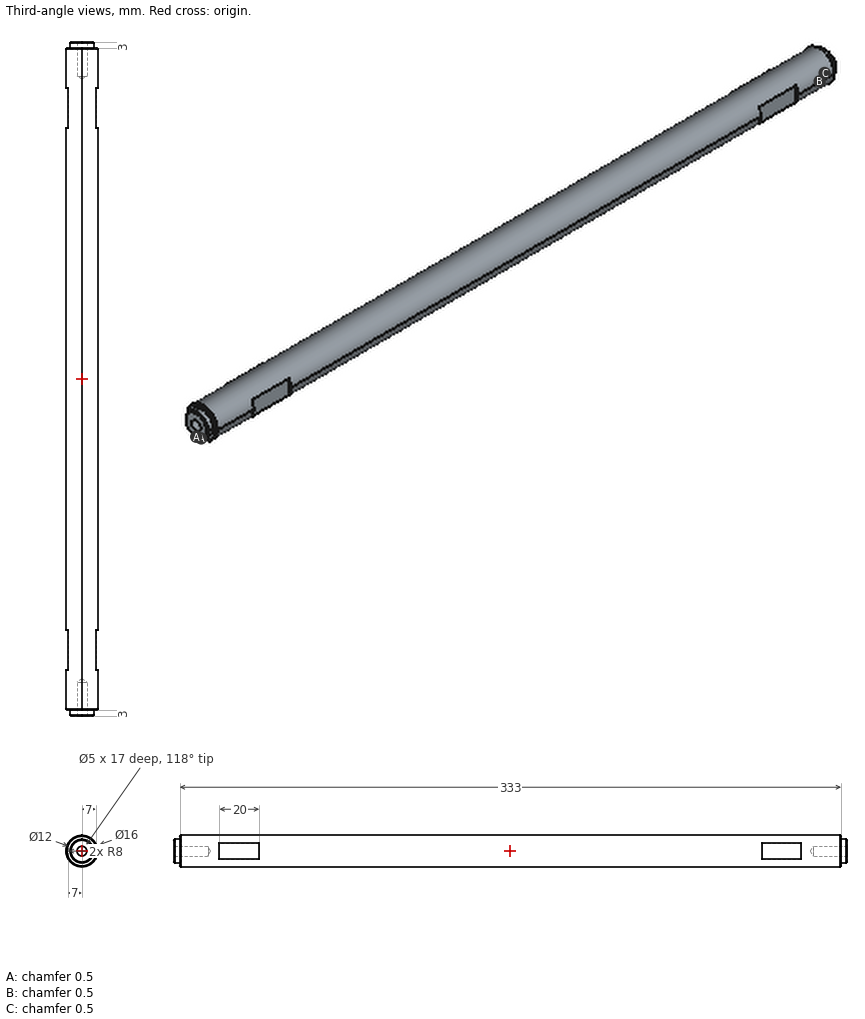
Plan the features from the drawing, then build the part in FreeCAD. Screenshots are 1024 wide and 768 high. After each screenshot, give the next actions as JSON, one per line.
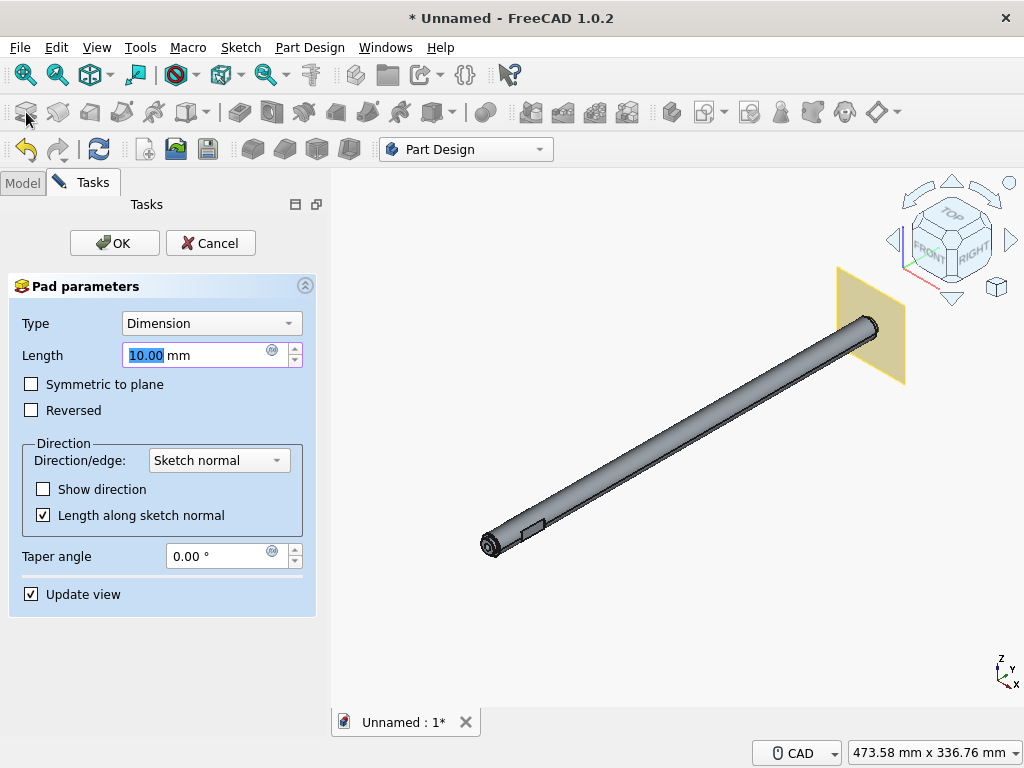
{"action": "type", "text": "3"}
{"action": "key", "text": "Tab"}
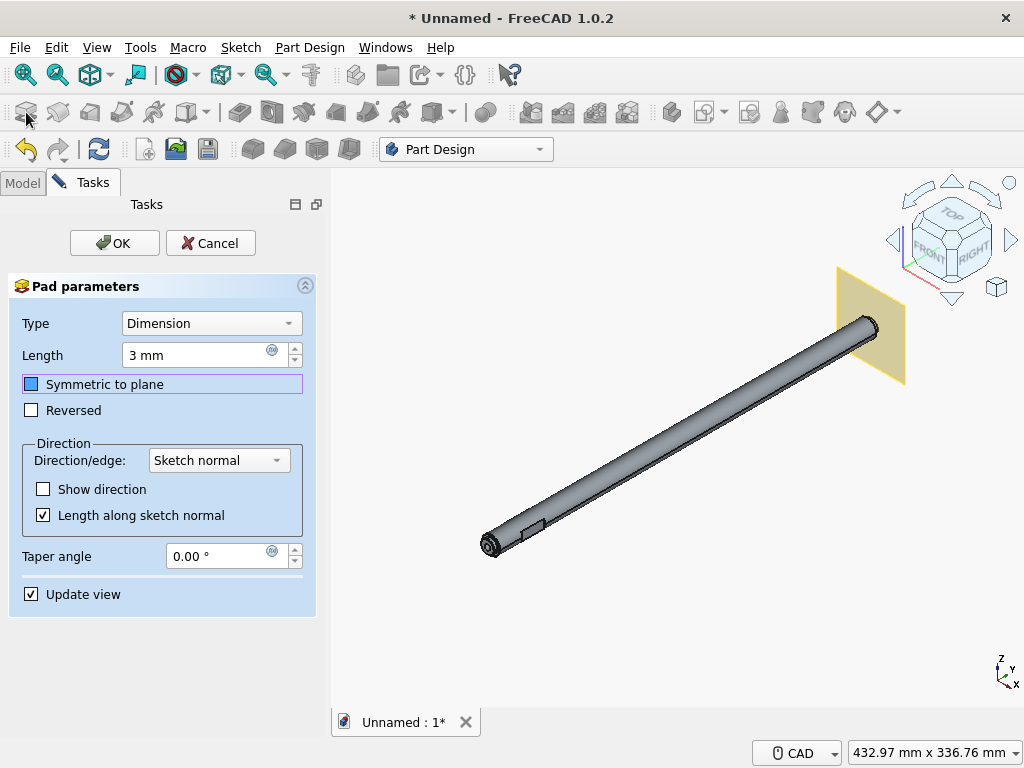
{"action": "left_click", "coordinate": [115, 243]}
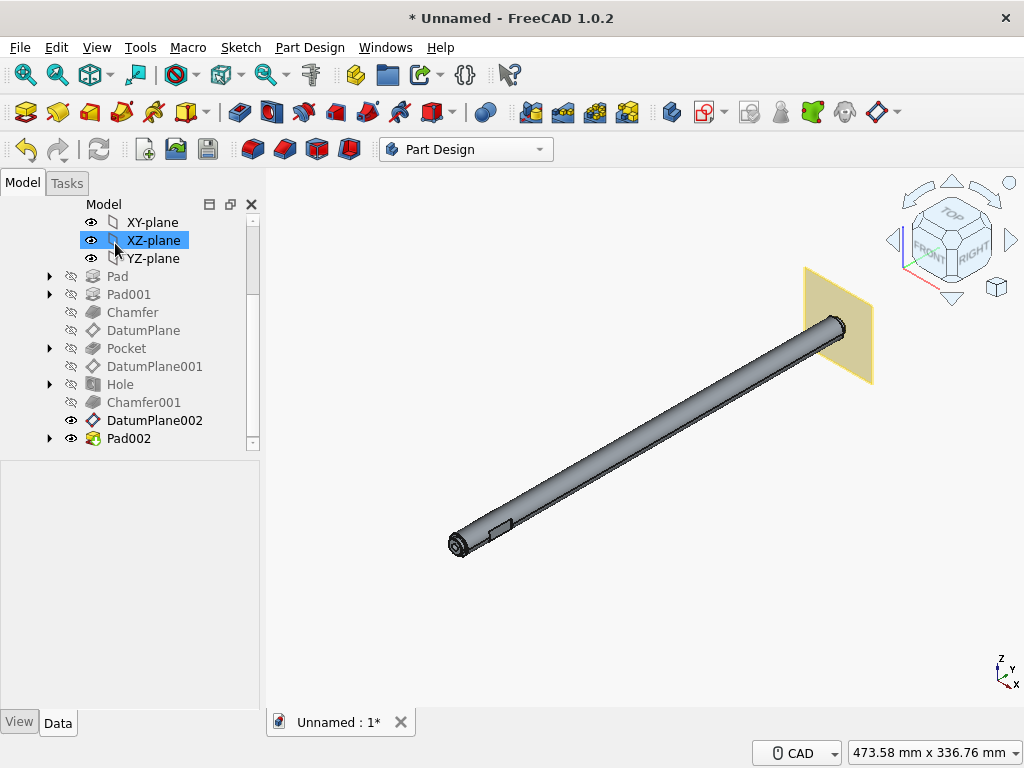
{"action": "left_click", "coordinate": [116, 420]}
{"action": "key", "text": "space"}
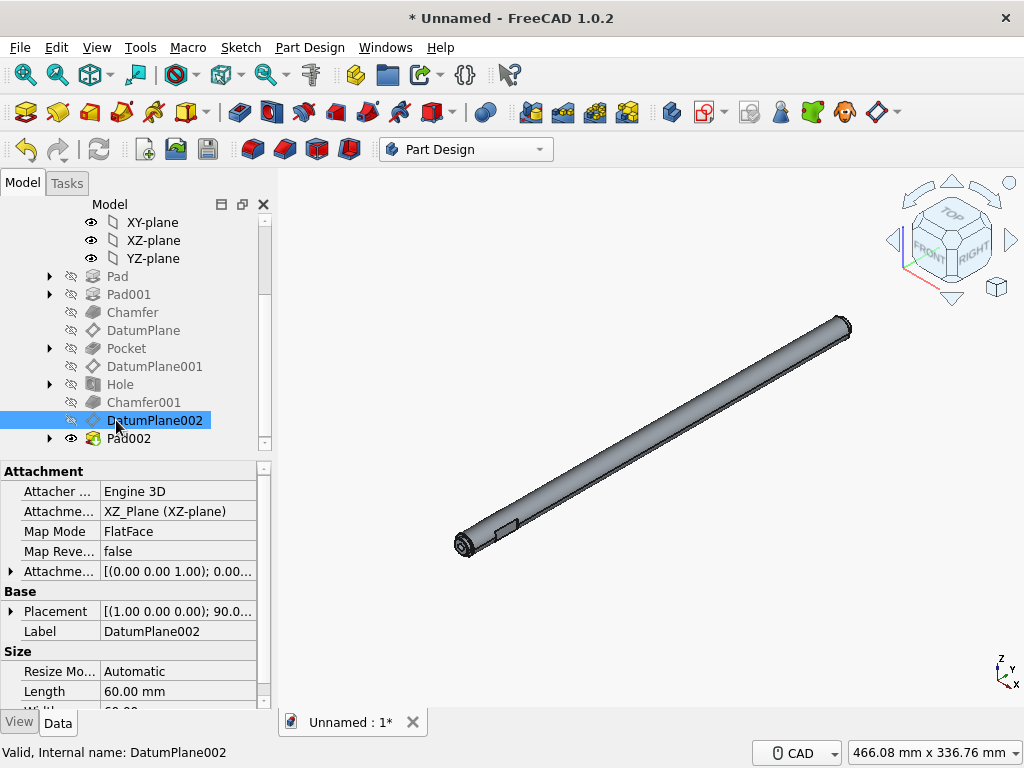
{"action": "key", "text": "2"}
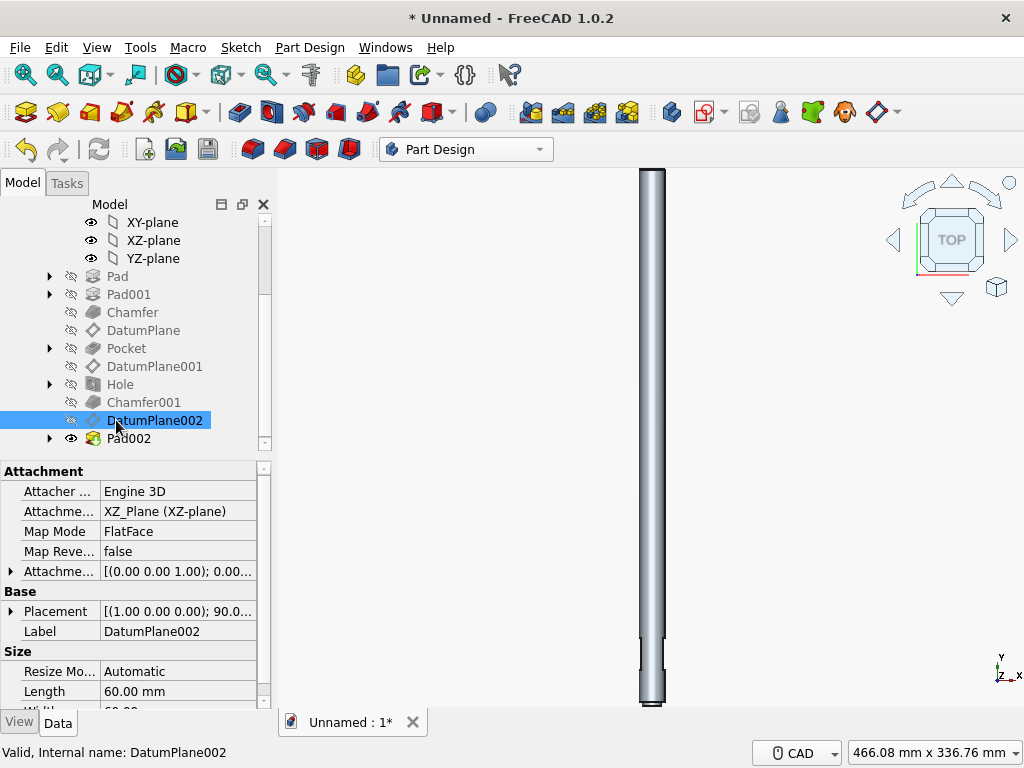
{"action": "left_click", "coordinate": [26, 76]}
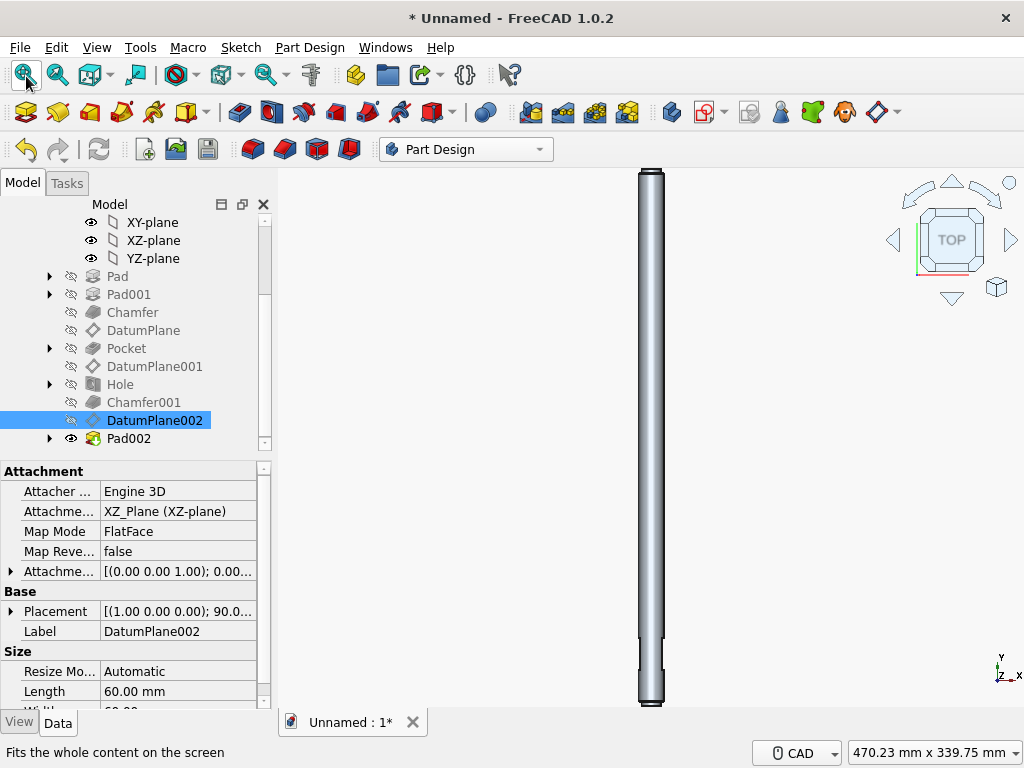
{"action": "key", "text": "0"}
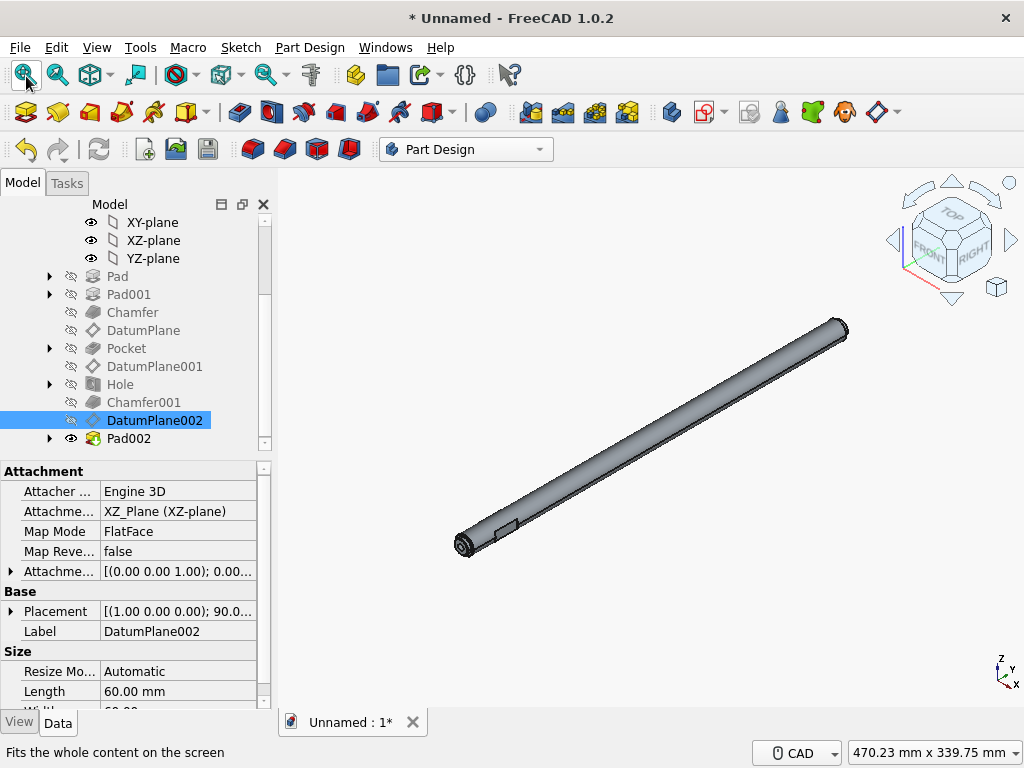
{"action": "key", "text": "1"}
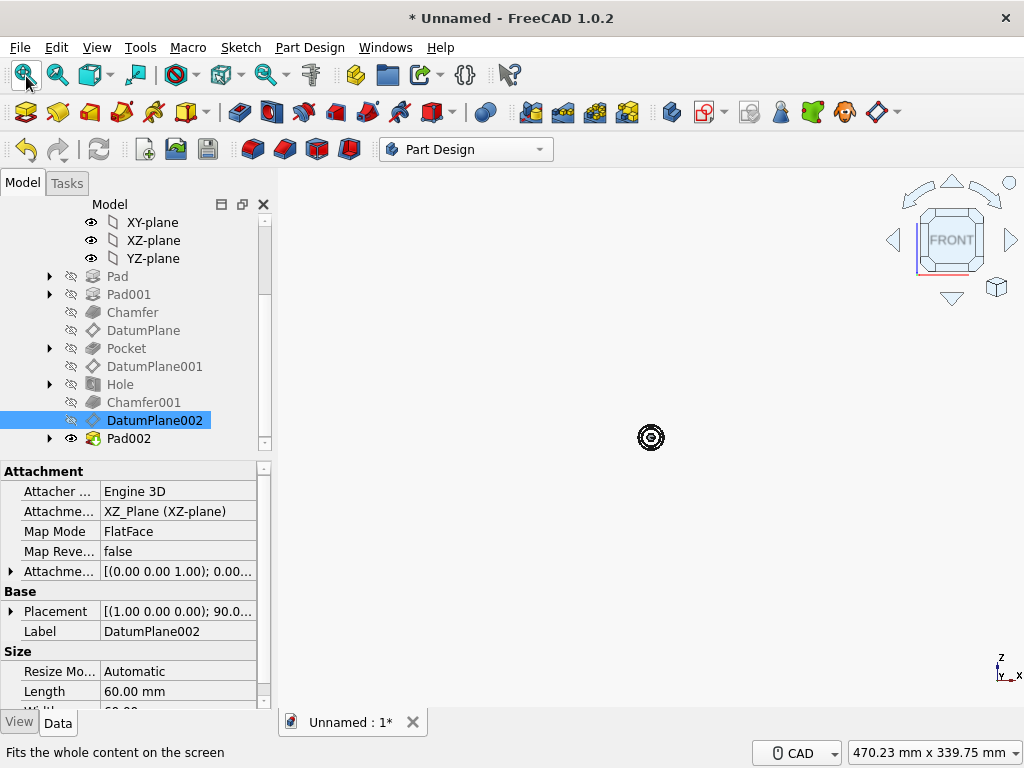
{"action": "key", "text": "v f"}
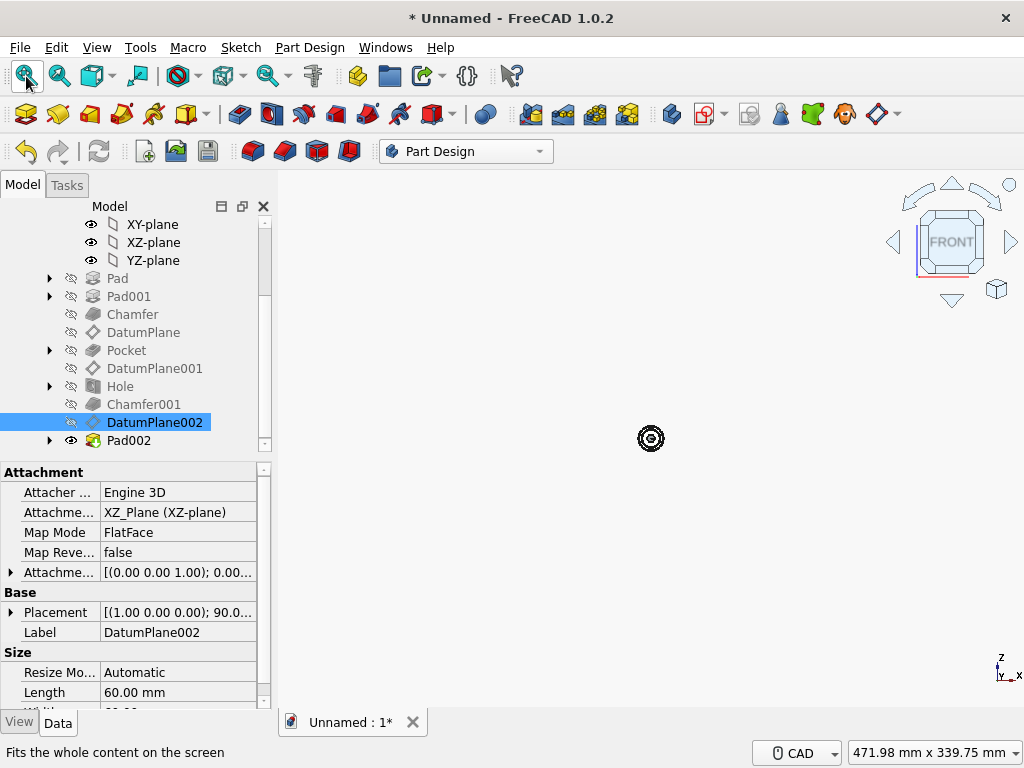
{"action": "key", "text": "3"}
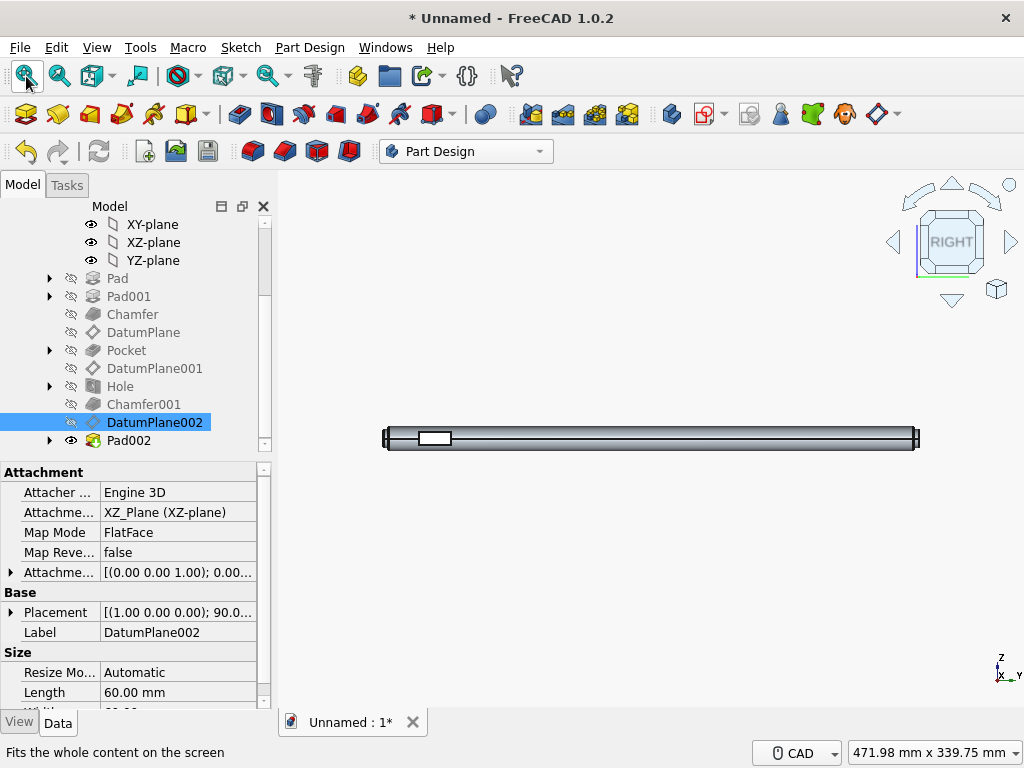
{"action": "key", "text": "5"}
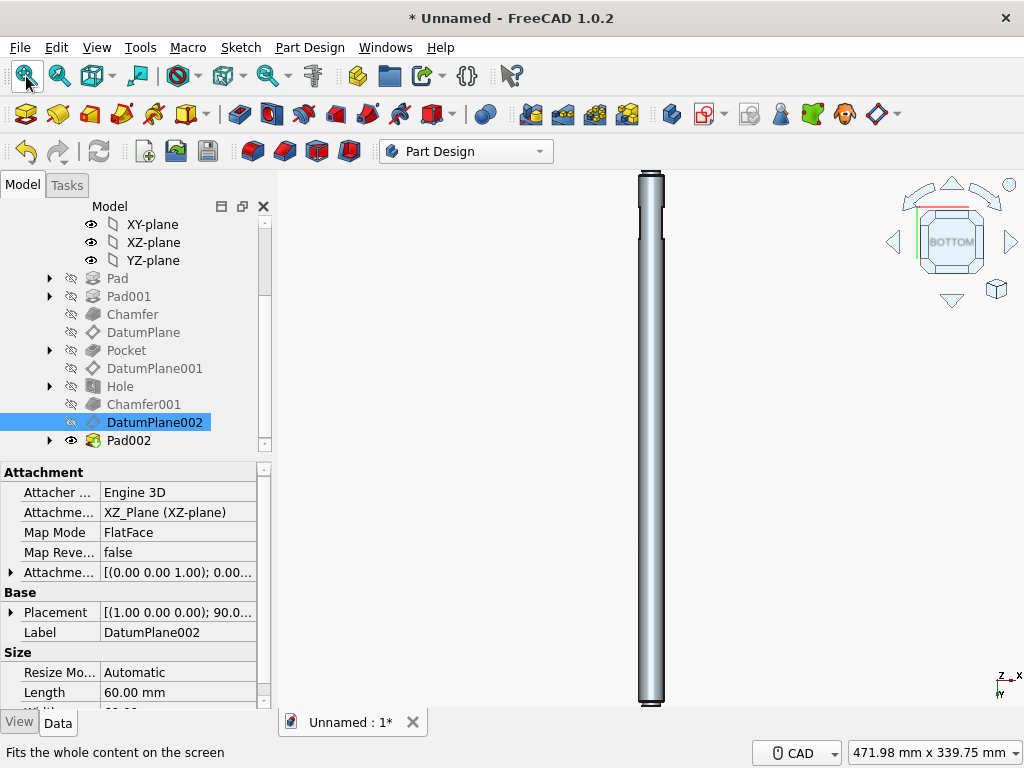
{"action": "key", "text": "4"}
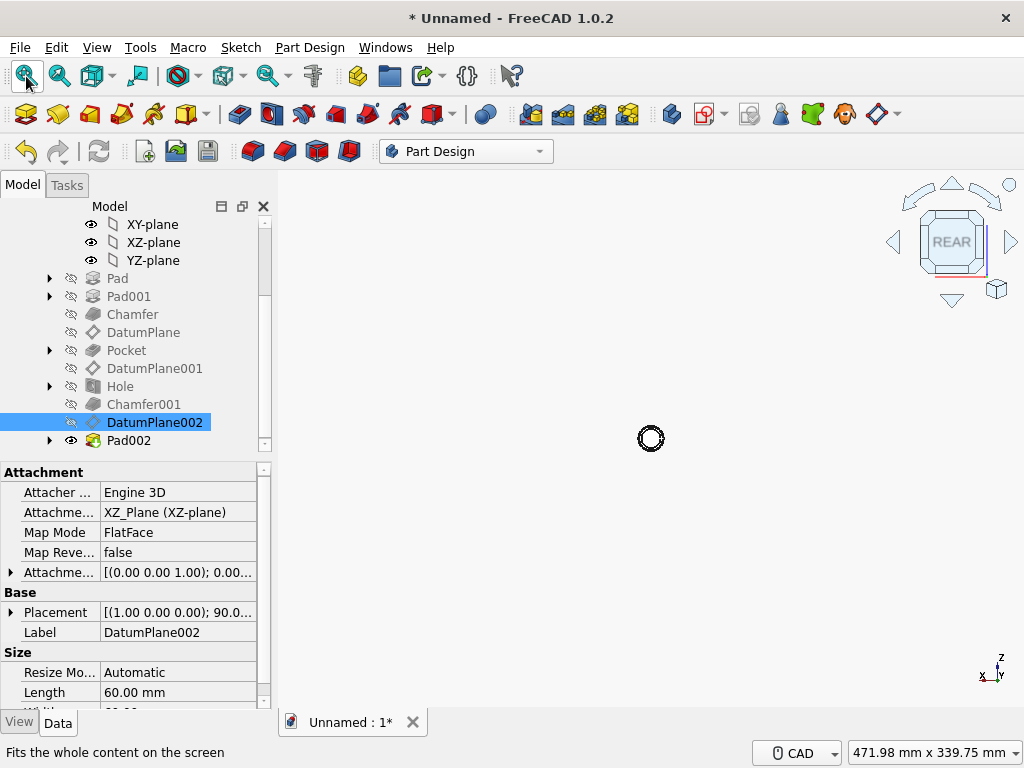
{"action": "key", "text": "v f"}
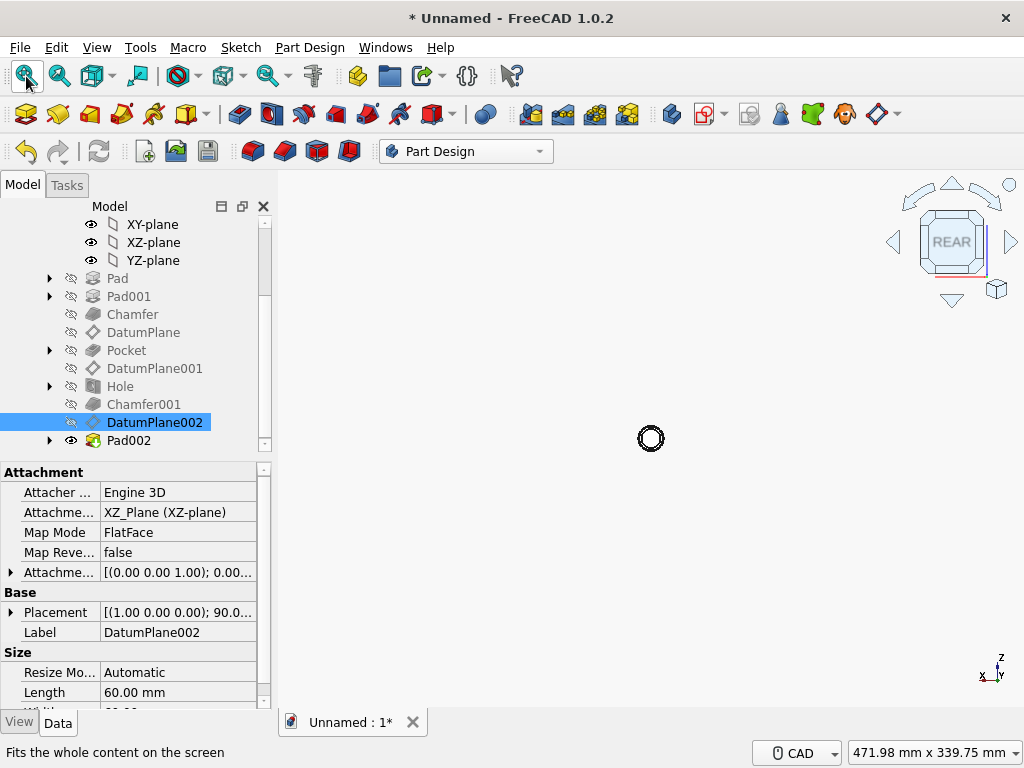
{"action": "left_click", "coordinate": [660, 438]}